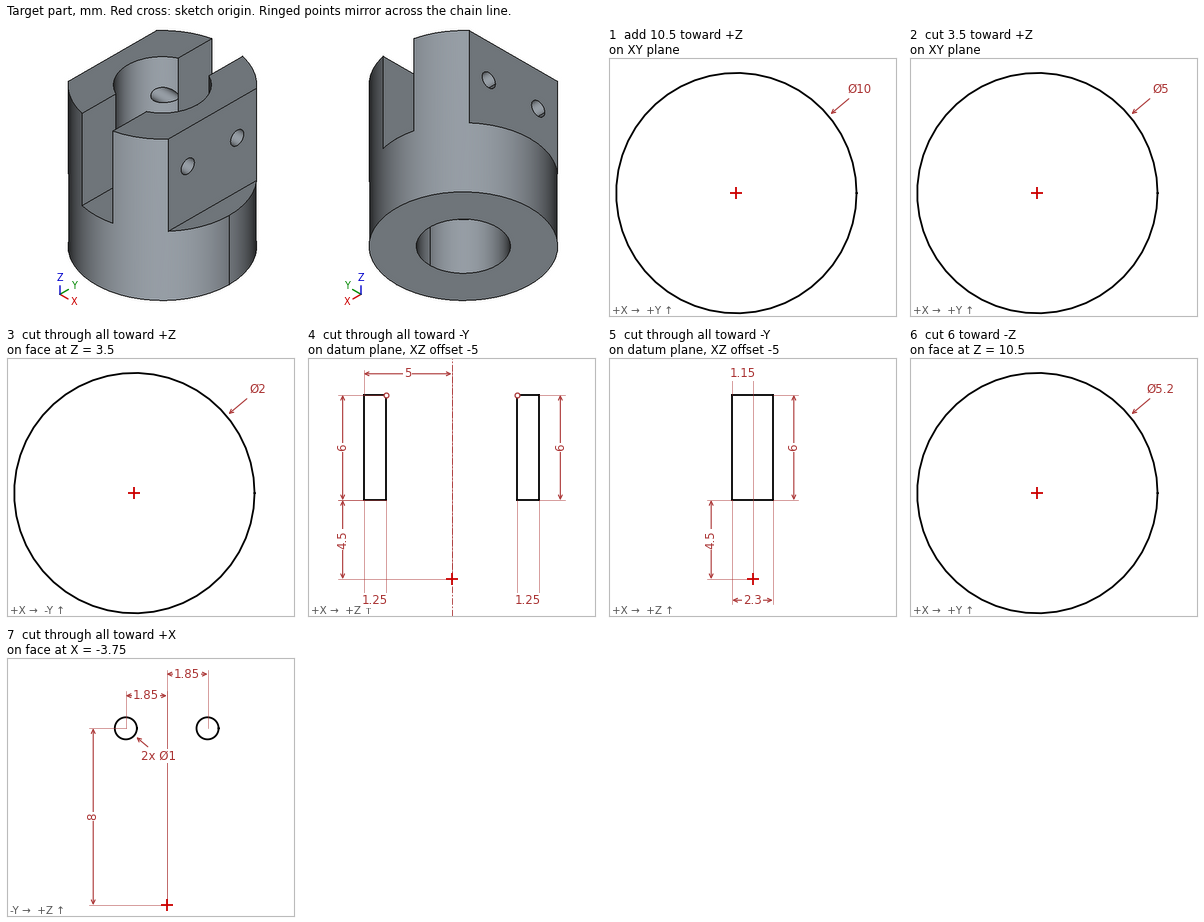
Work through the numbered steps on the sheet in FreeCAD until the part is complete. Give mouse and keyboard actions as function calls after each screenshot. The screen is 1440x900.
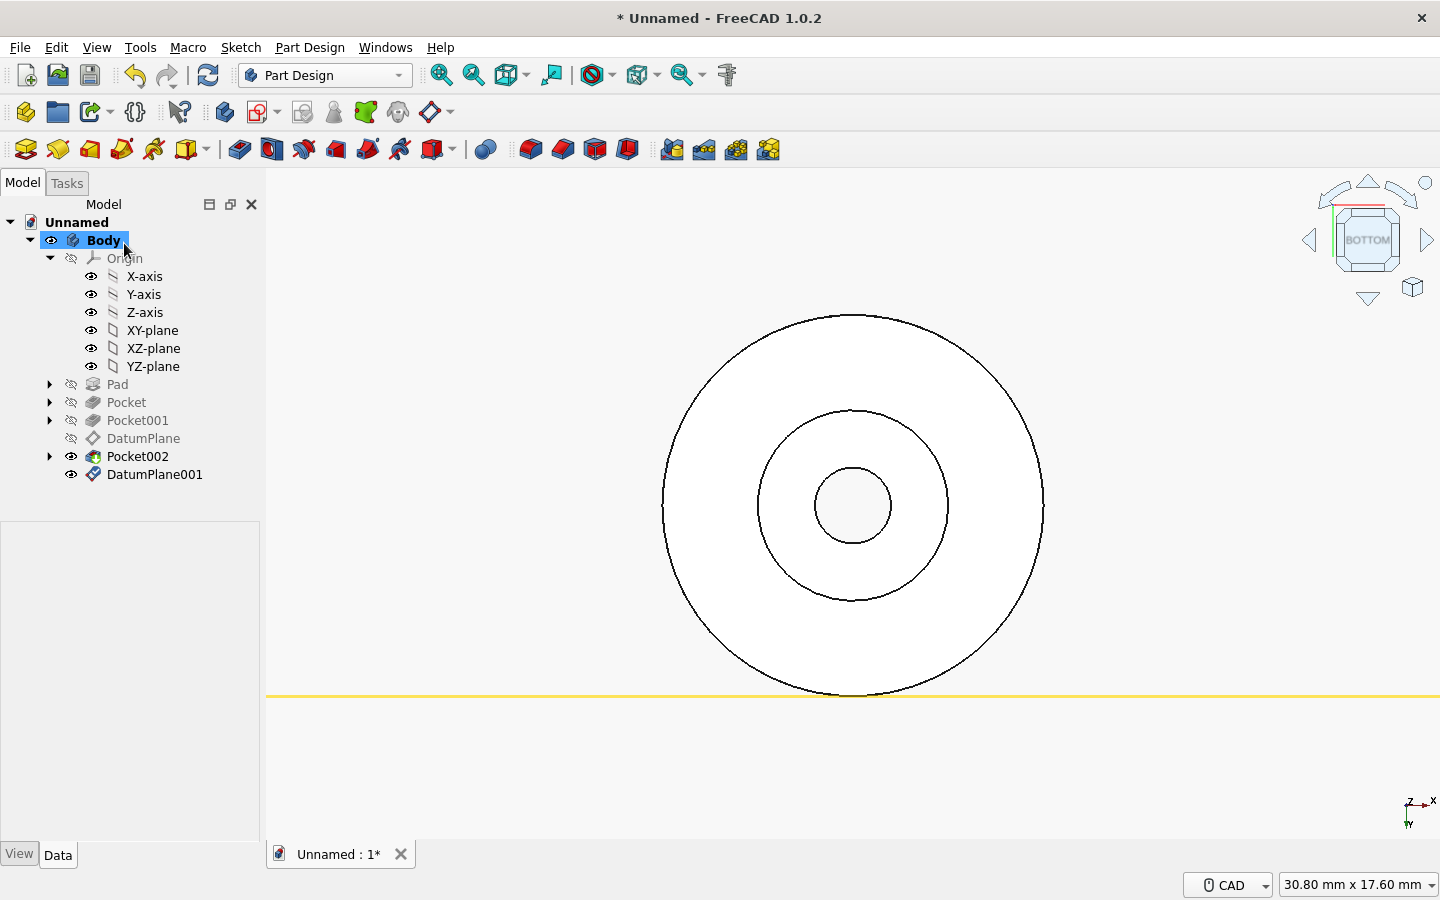
click(116, 474)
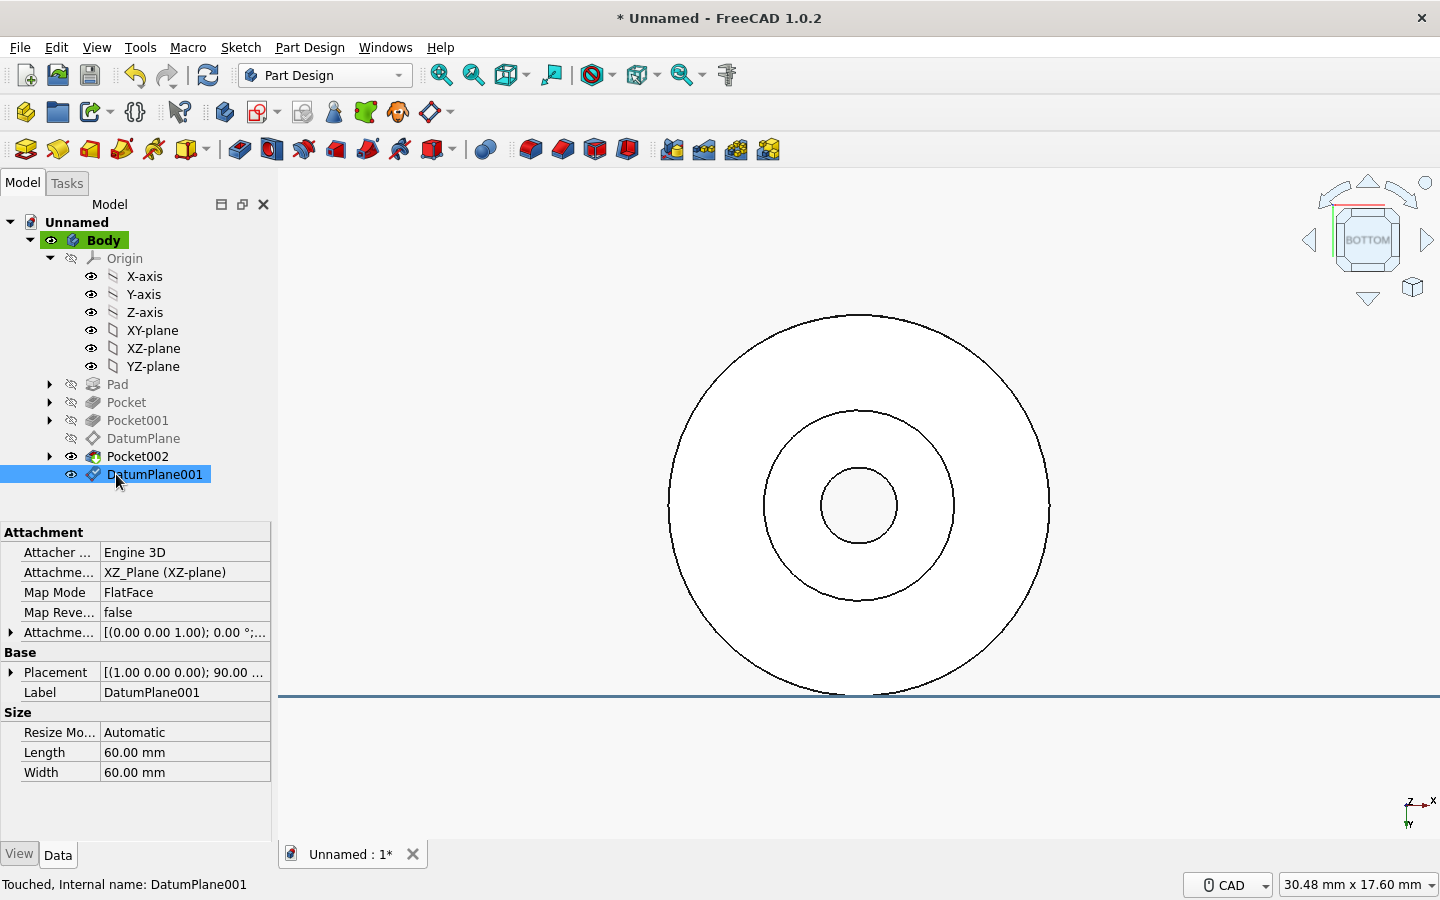
click(258, 112)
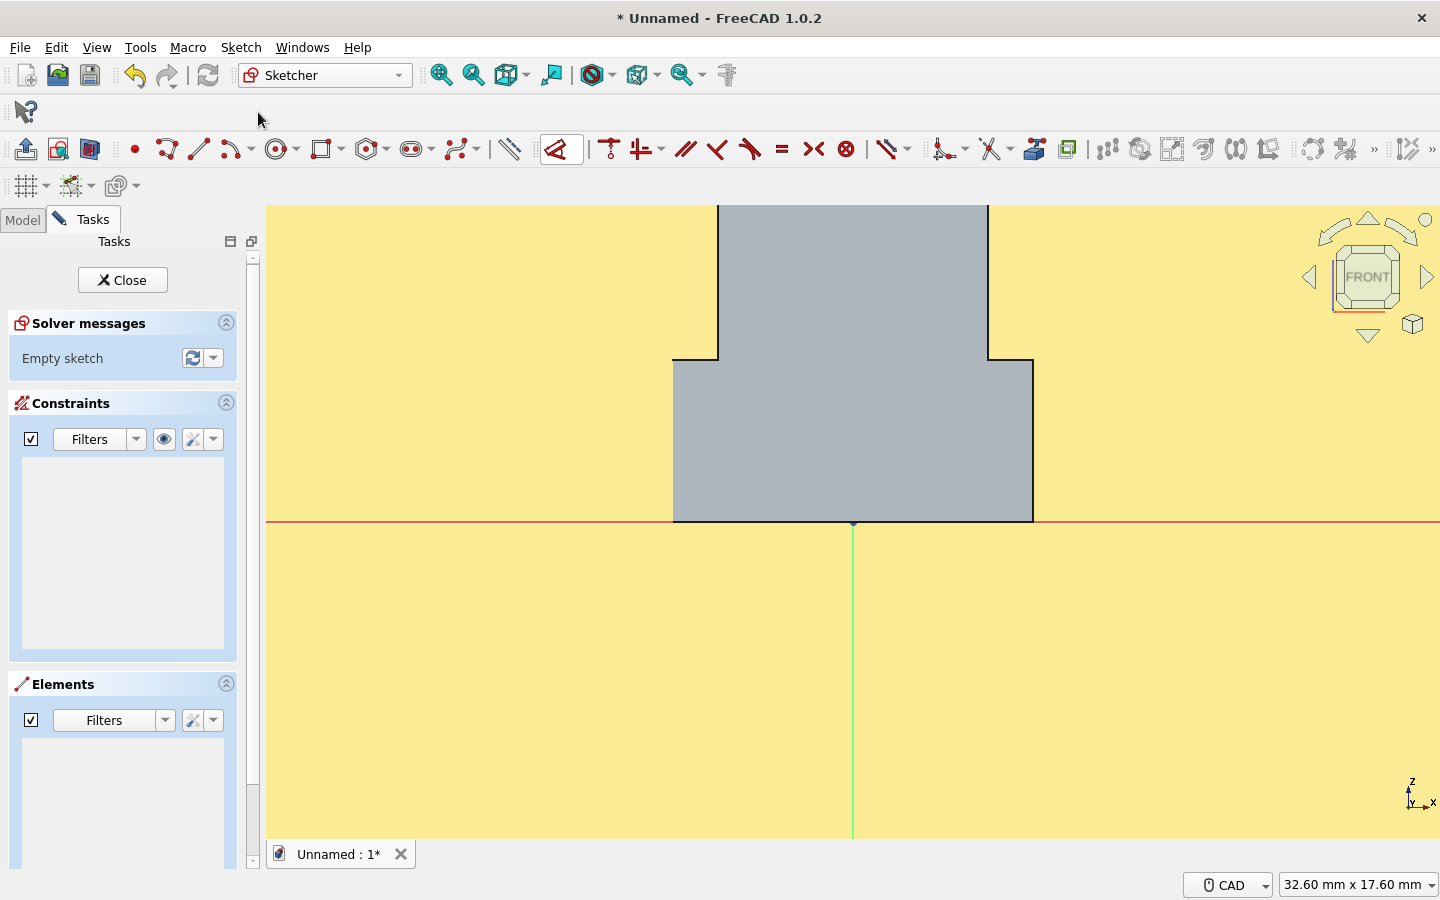
key(q)
key(s)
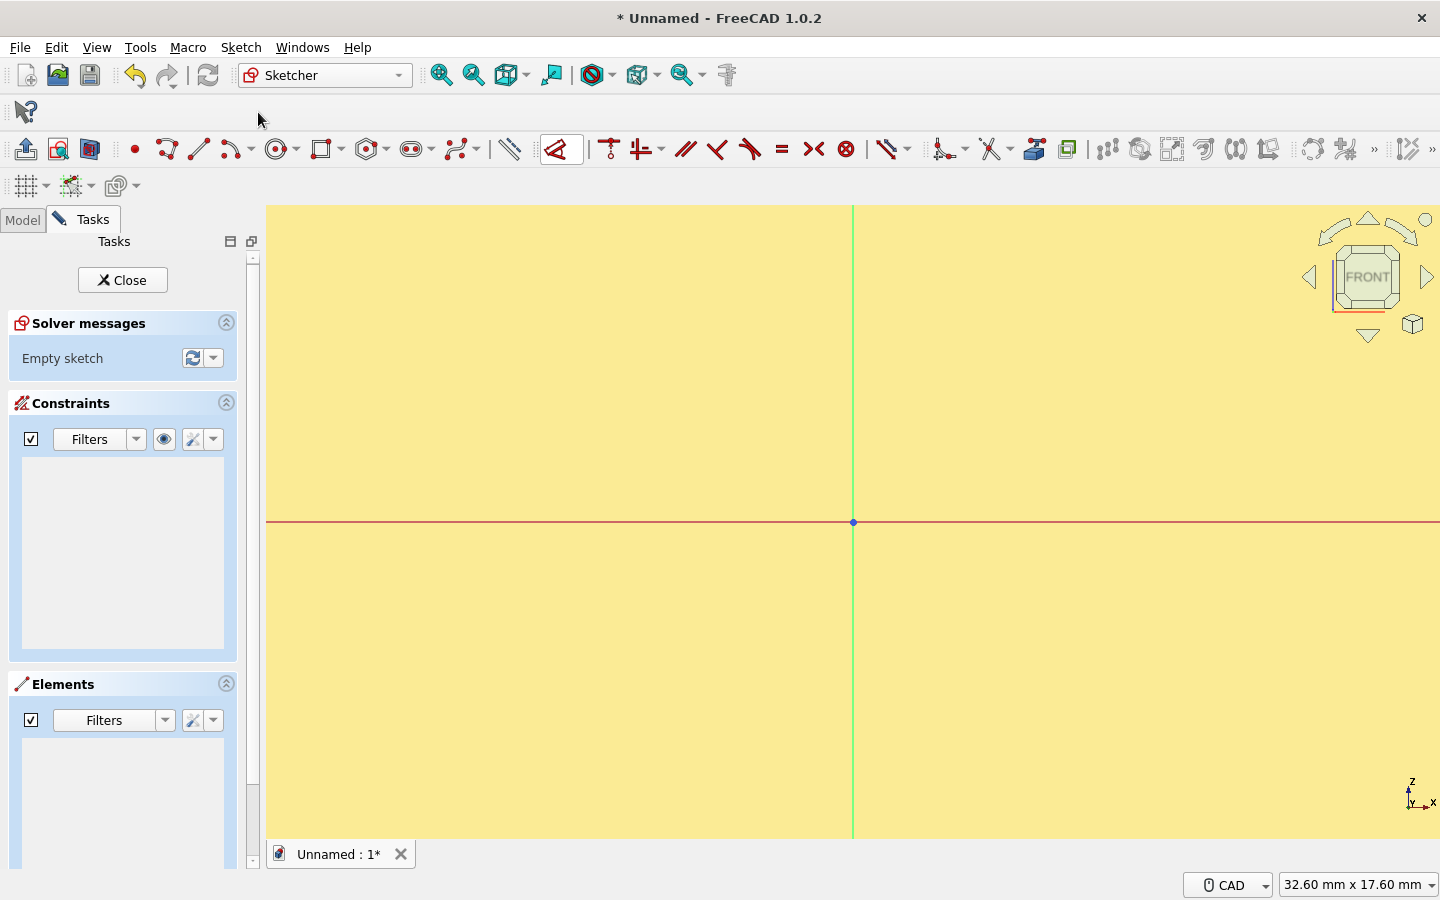
scroll(475, 811, down, 1)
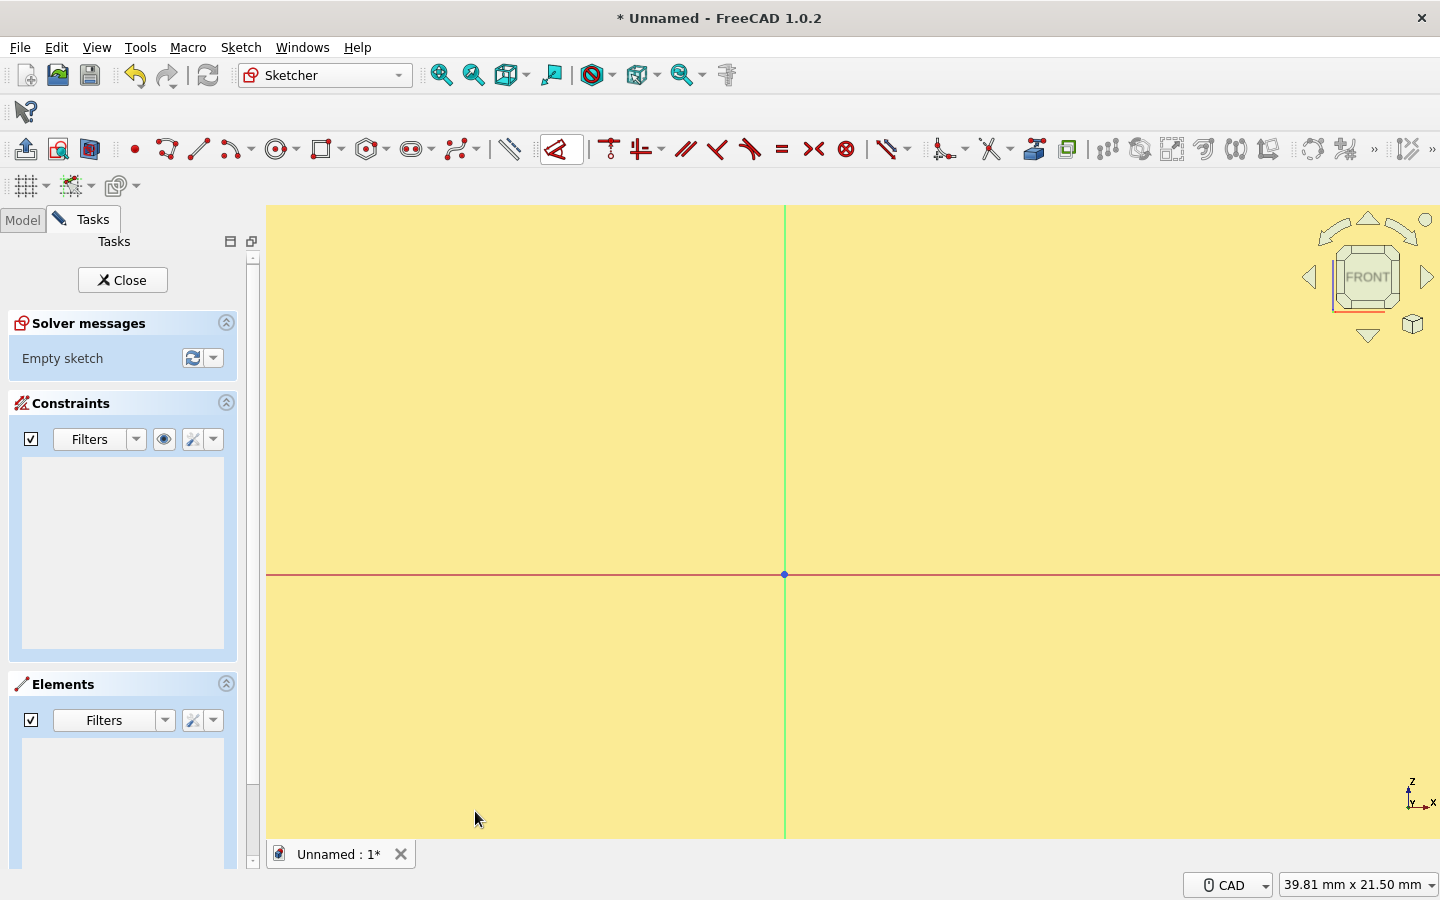
key(g)
key(r)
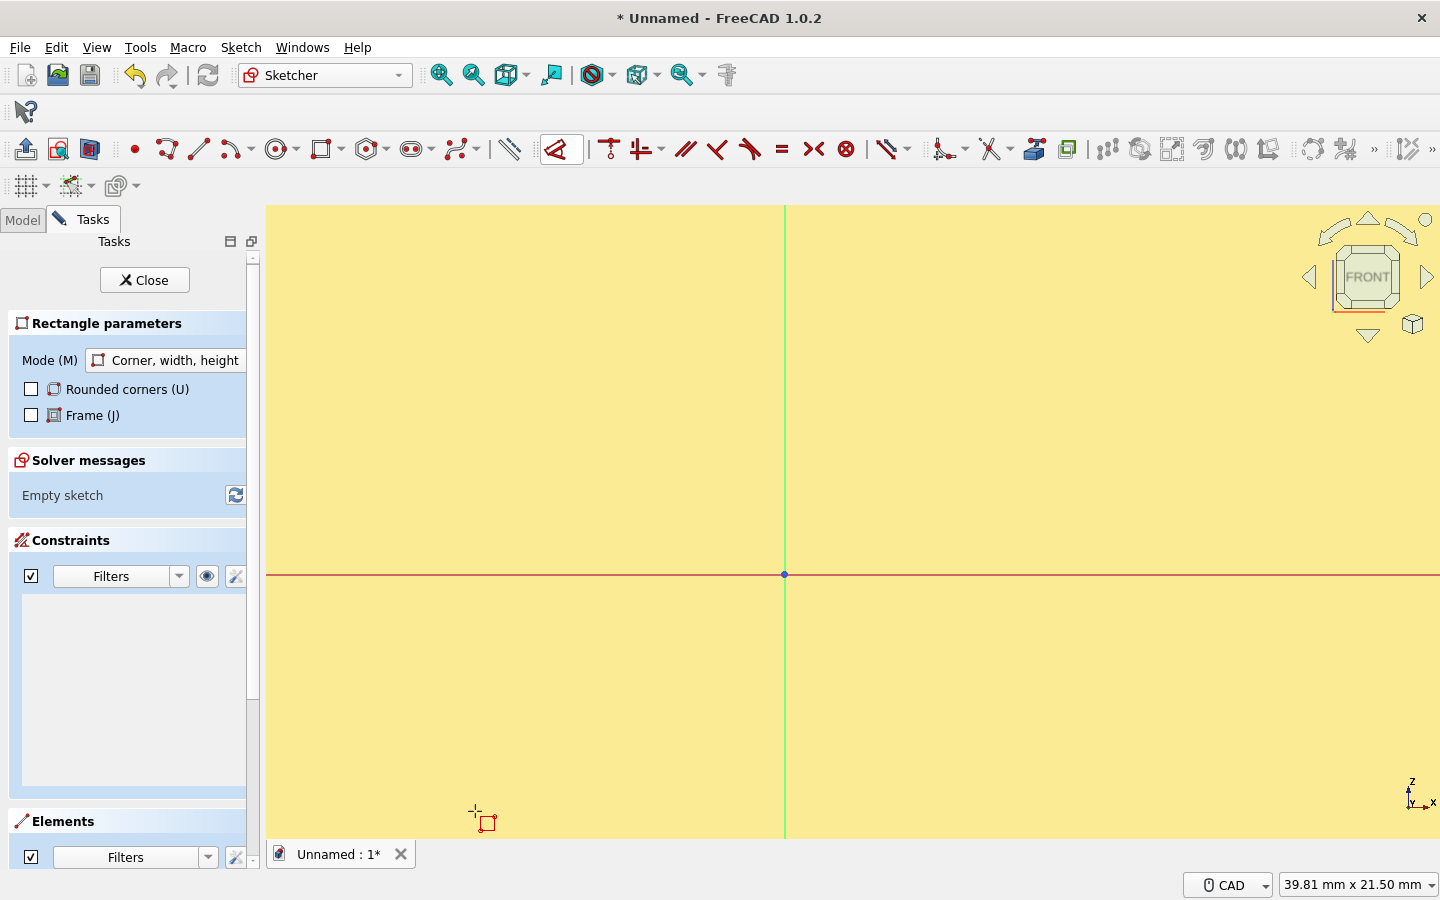
click(751, 265)
move(818, 442)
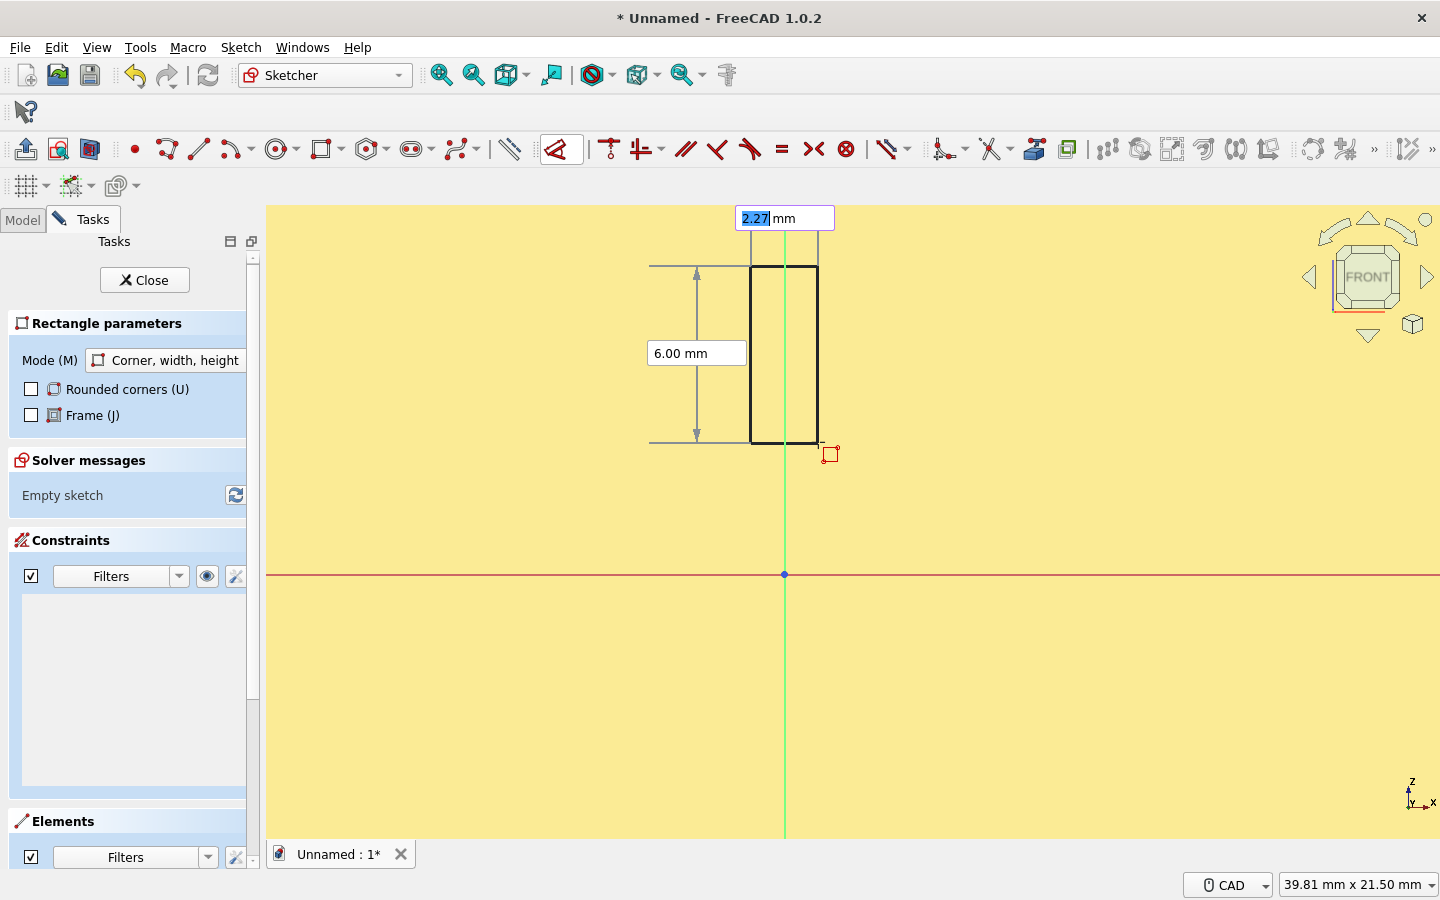
text(2.3)
key(Tab)
text(6)
key(Return)
key(Escape)